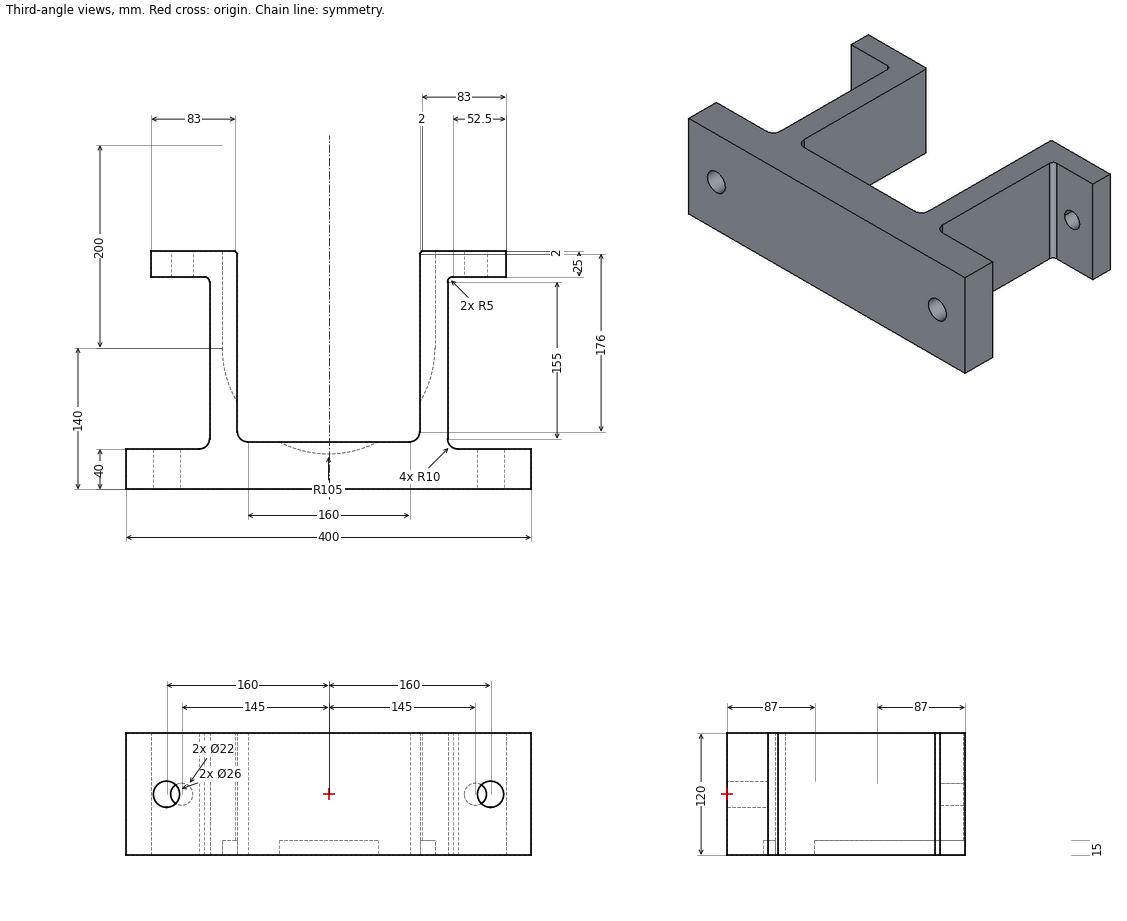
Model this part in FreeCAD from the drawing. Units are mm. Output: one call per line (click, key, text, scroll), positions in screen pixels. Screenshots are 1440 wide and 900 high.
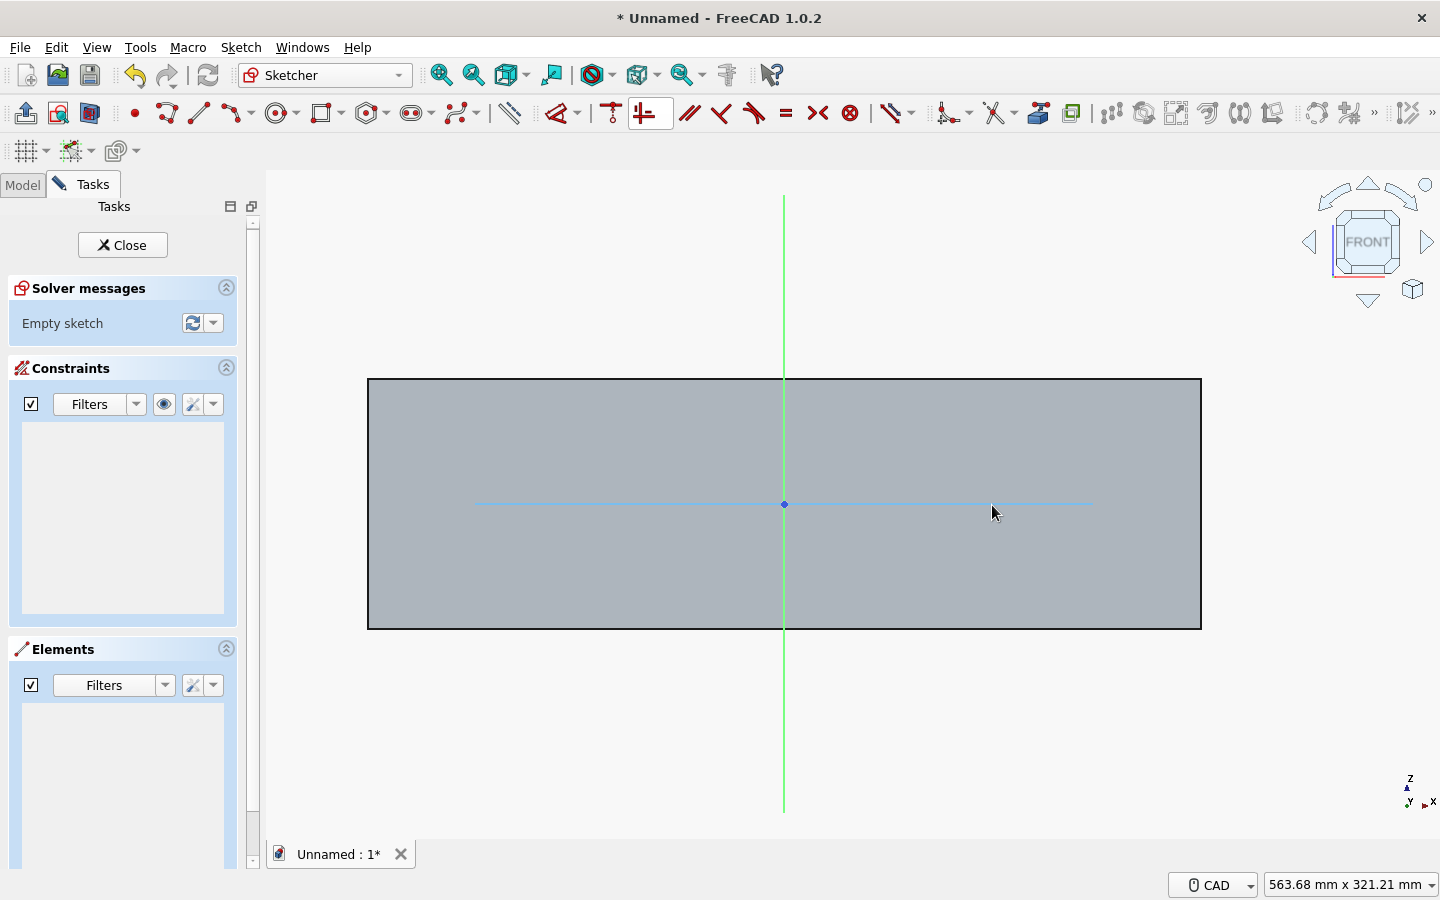
click(276, 114)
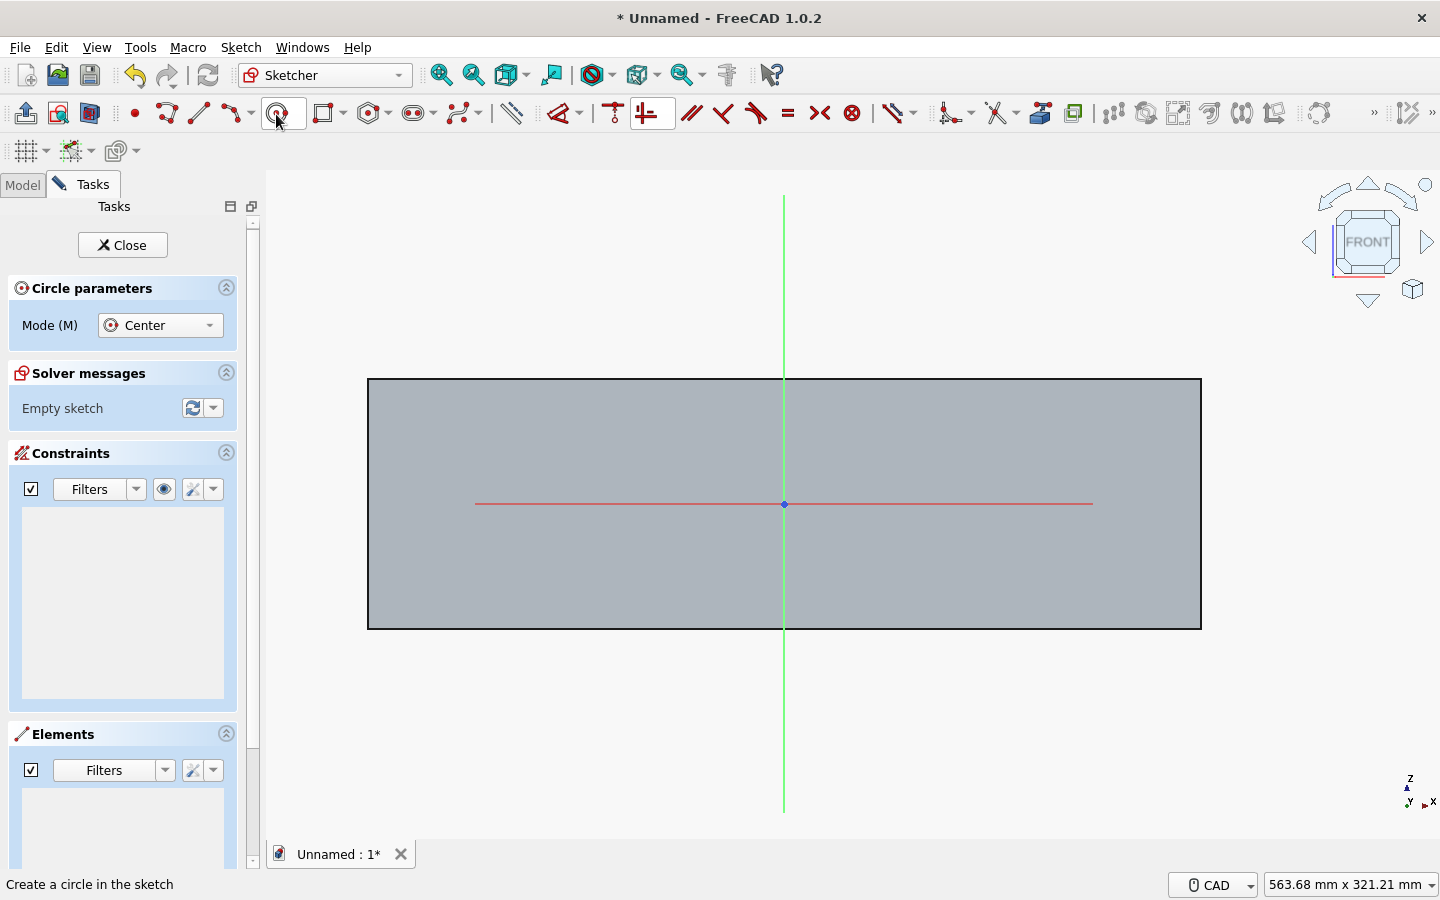
click(451, 504)
move(470, 485)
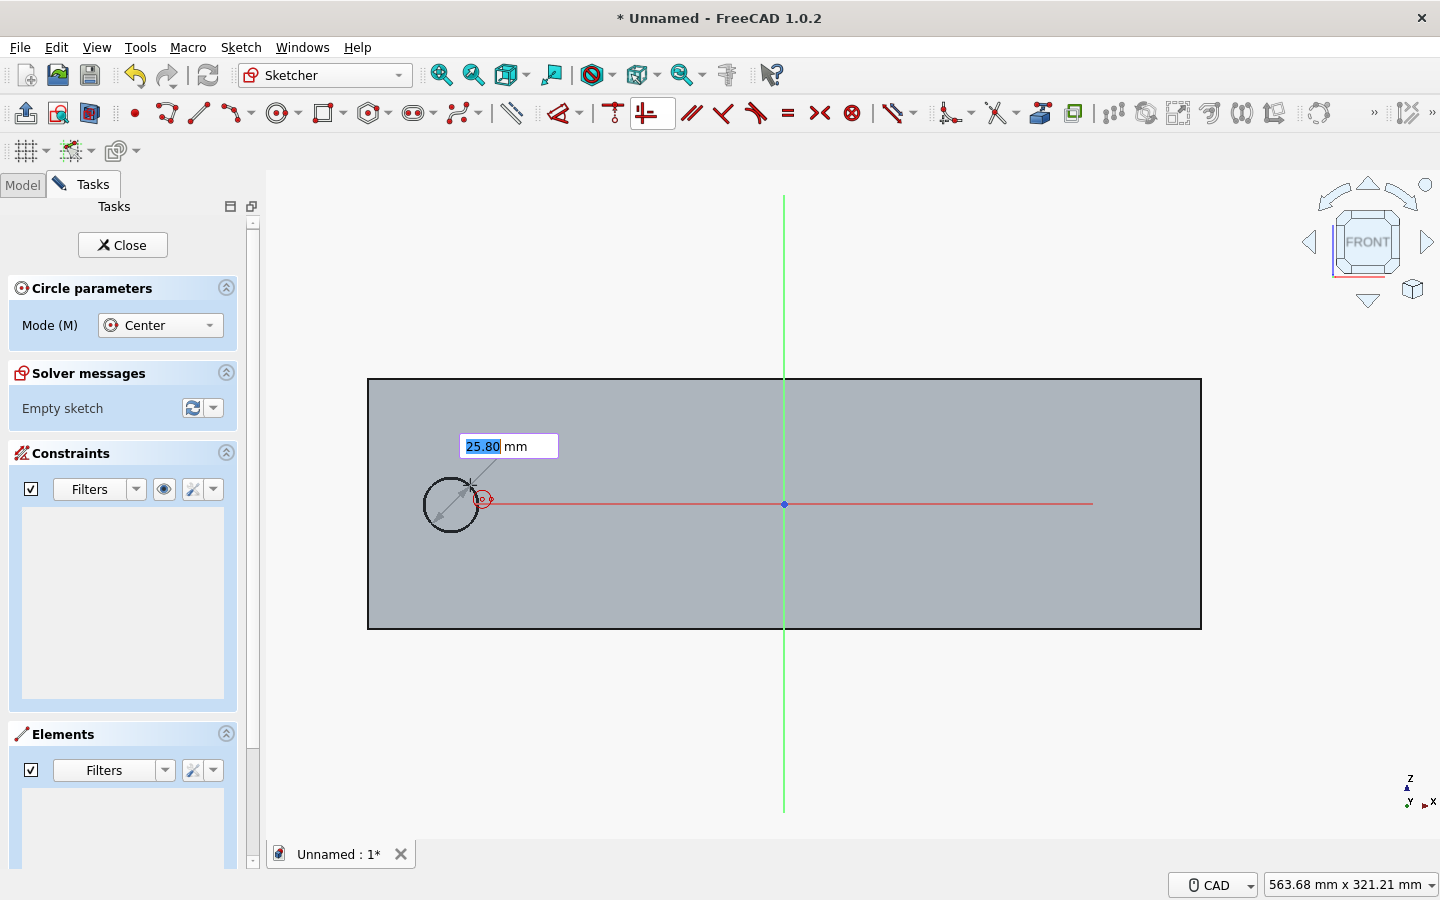
text(26)
key(Return)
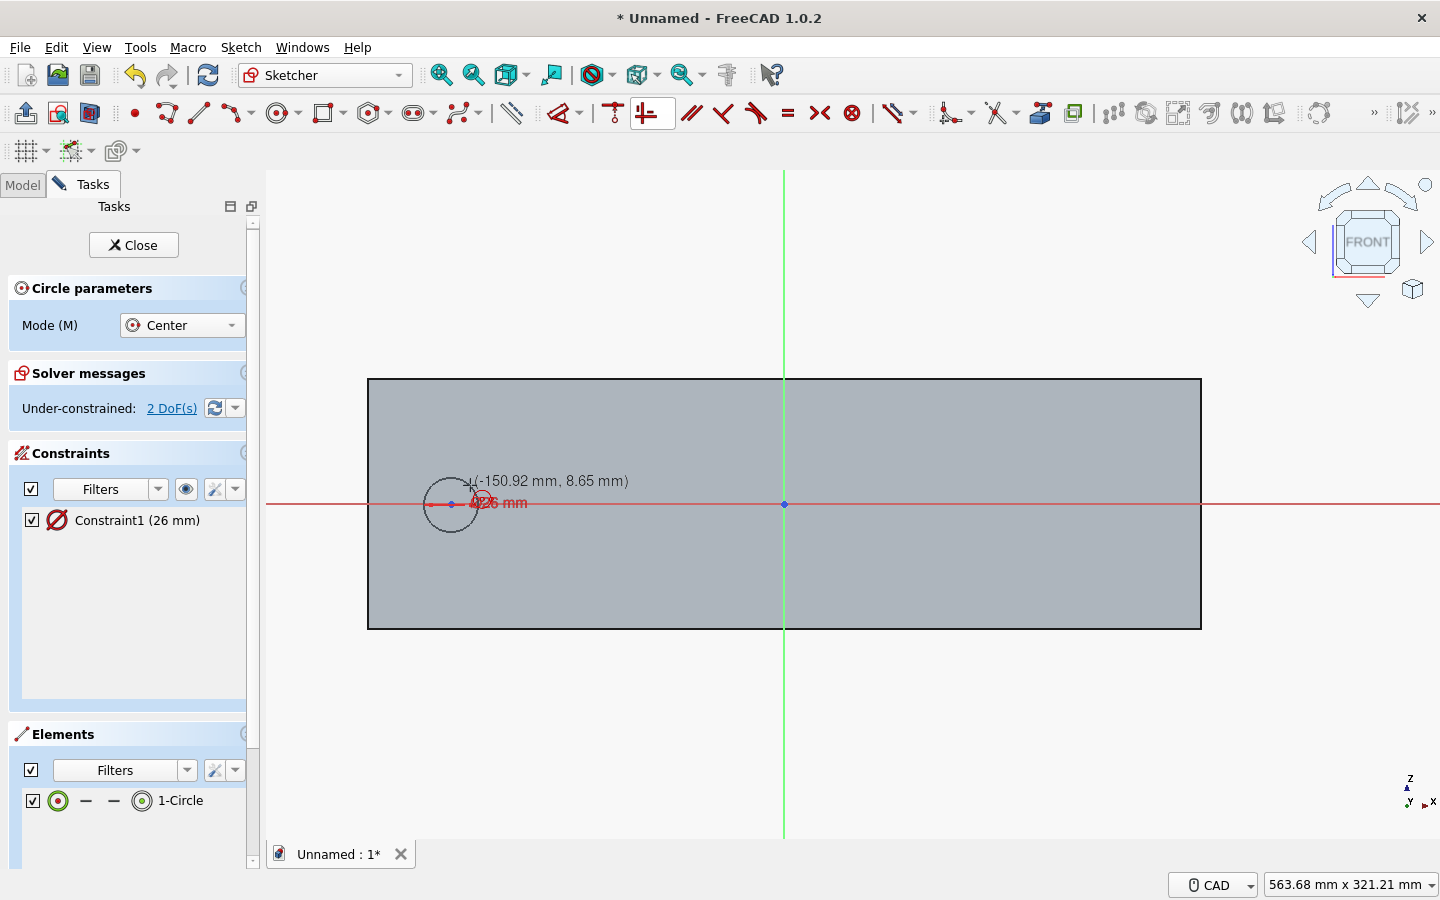
click(1118, 504)
move(1137, 485)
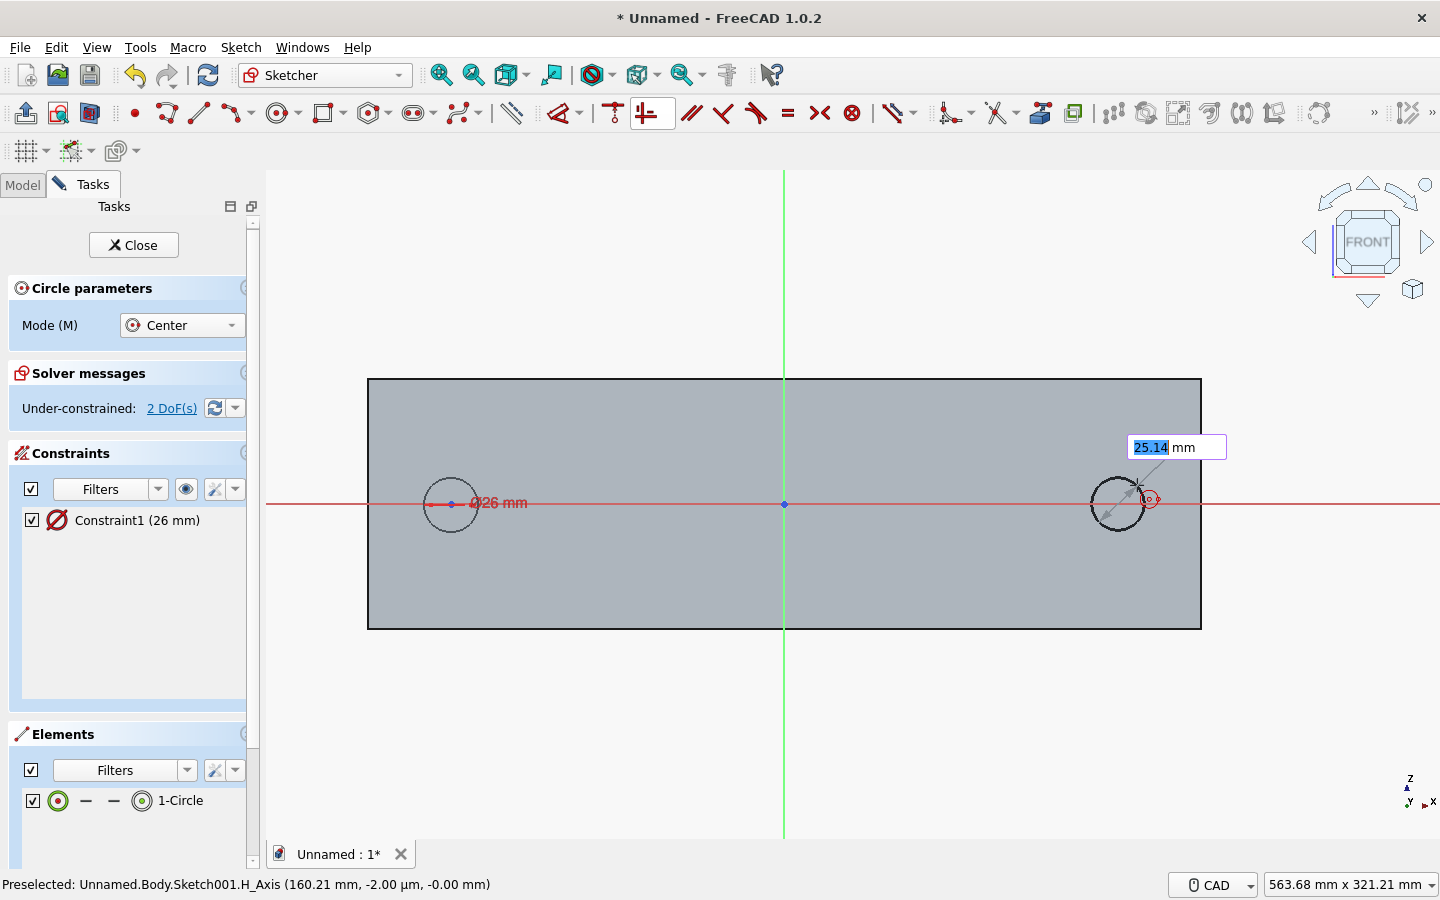
text(26)
key(Return)
key(Escape)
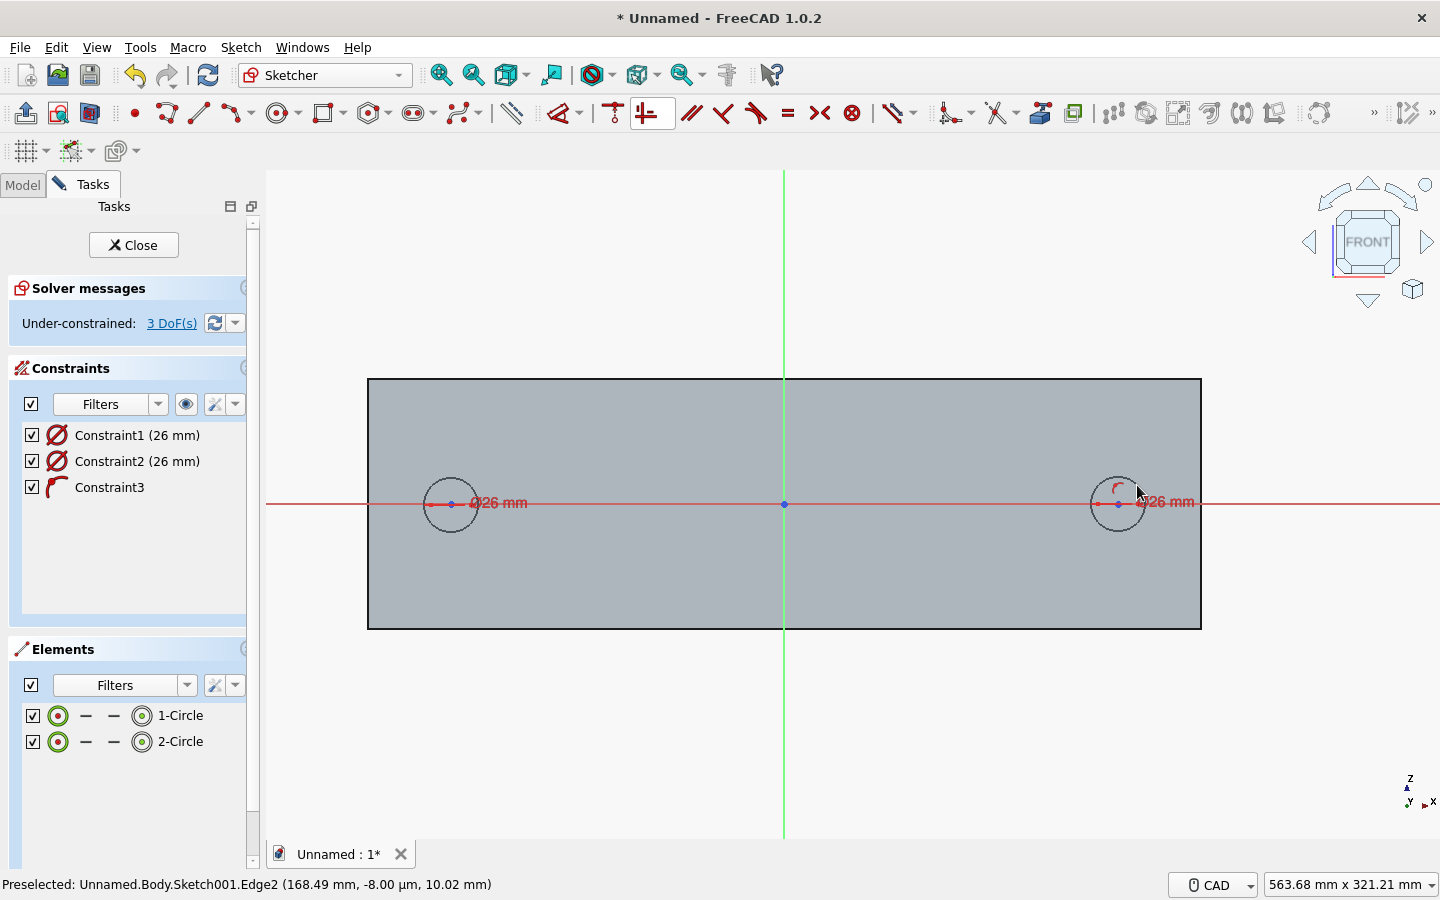
click(451, 505)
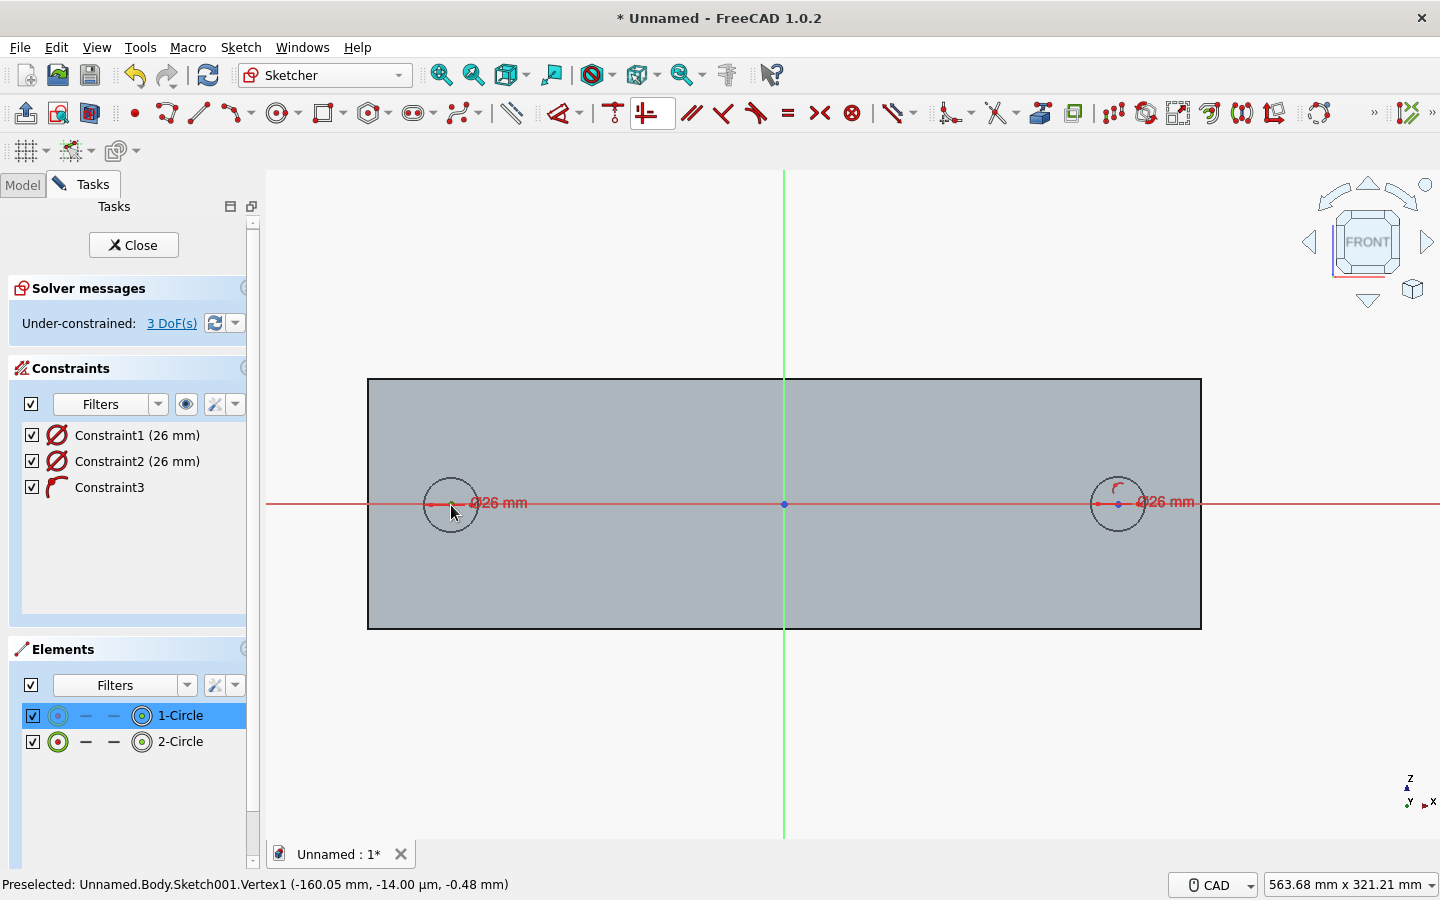
click(364, 504)